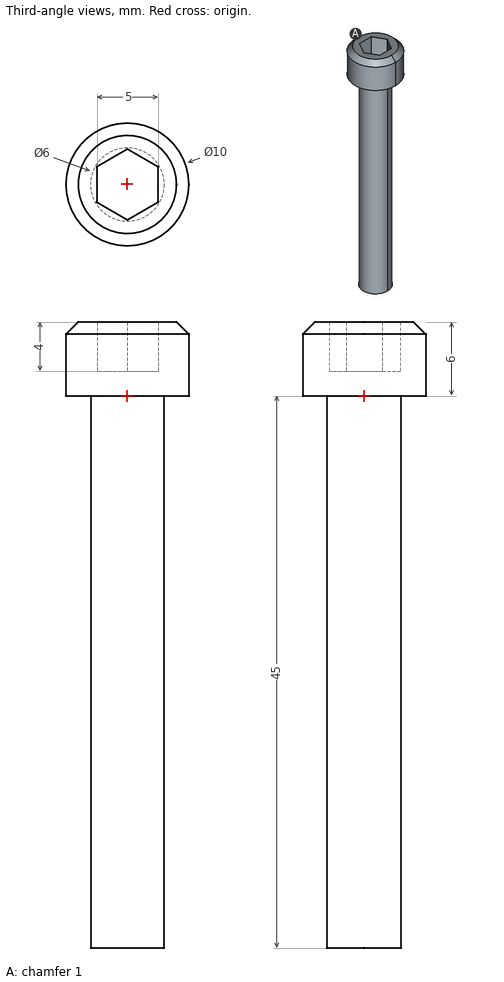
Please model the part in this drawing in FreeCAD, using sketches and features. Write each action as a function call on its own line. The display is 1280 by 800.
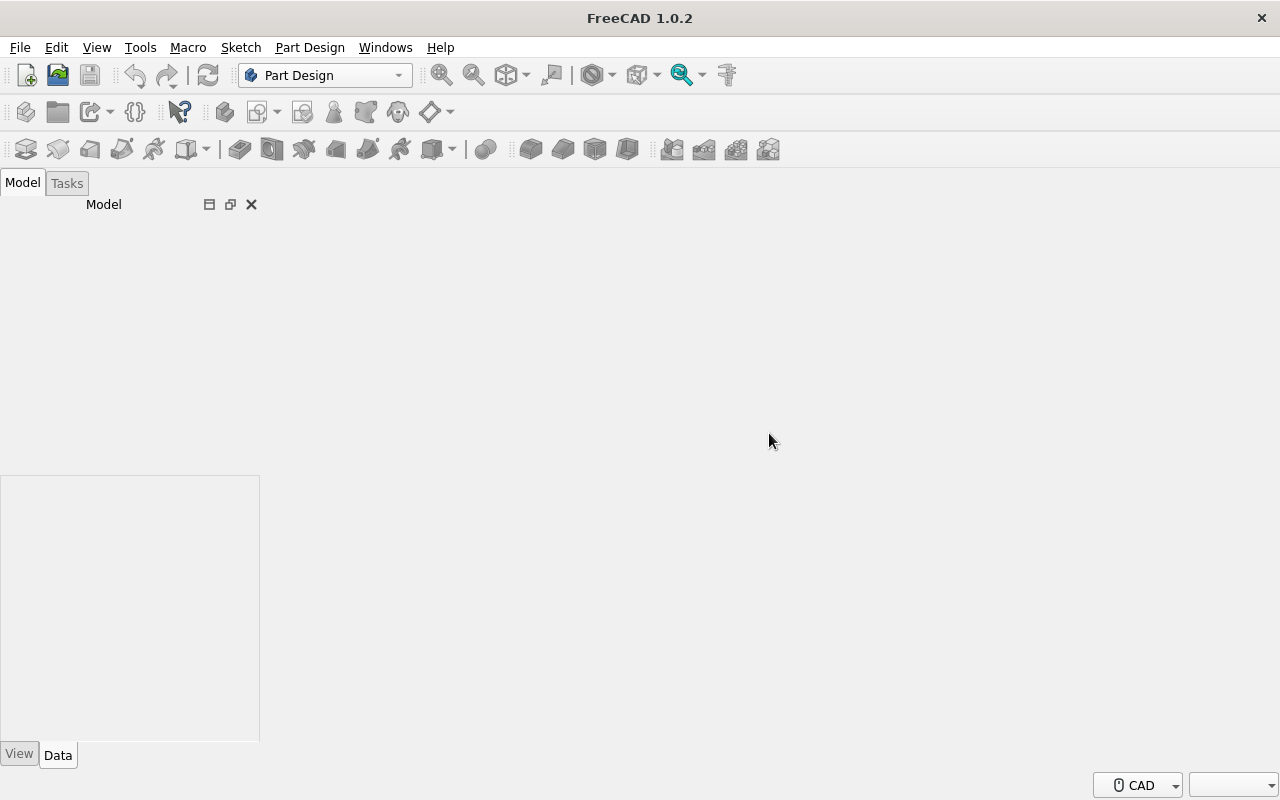
click(26, 76)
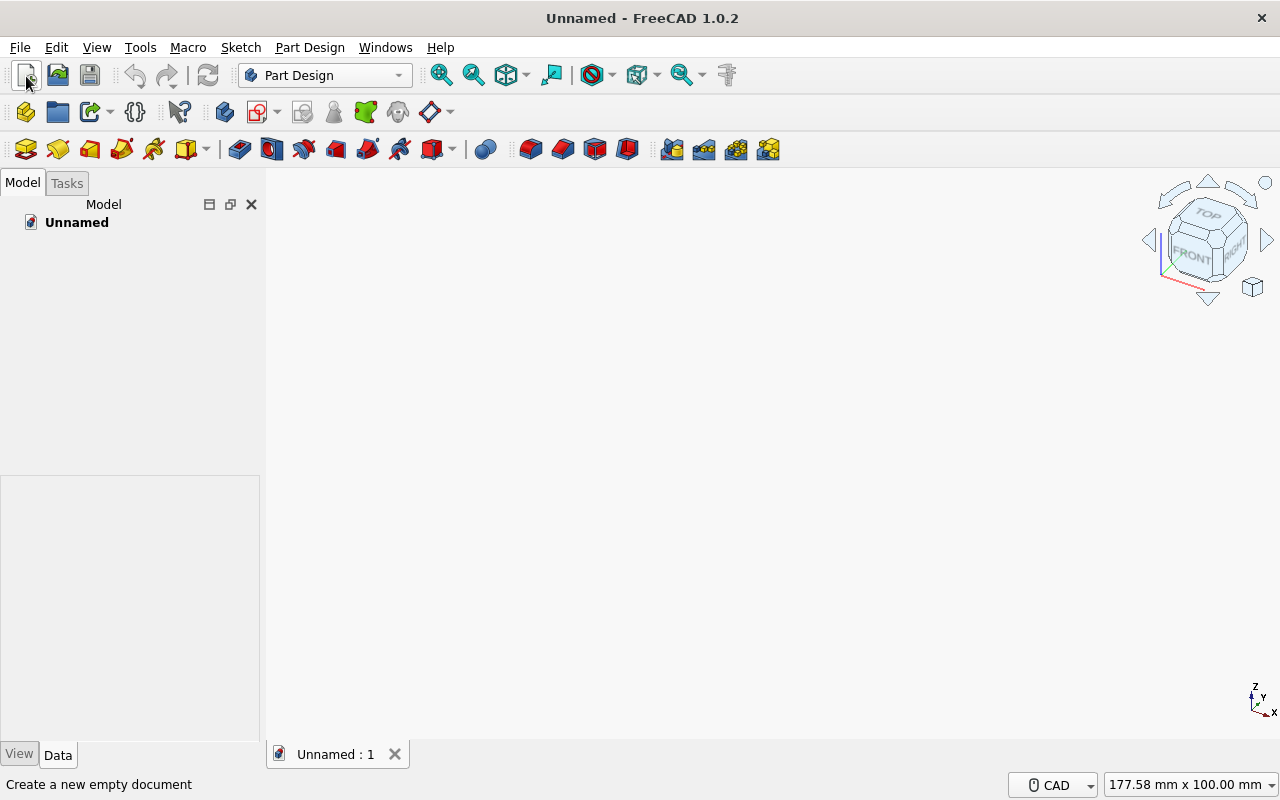
click(258, 112)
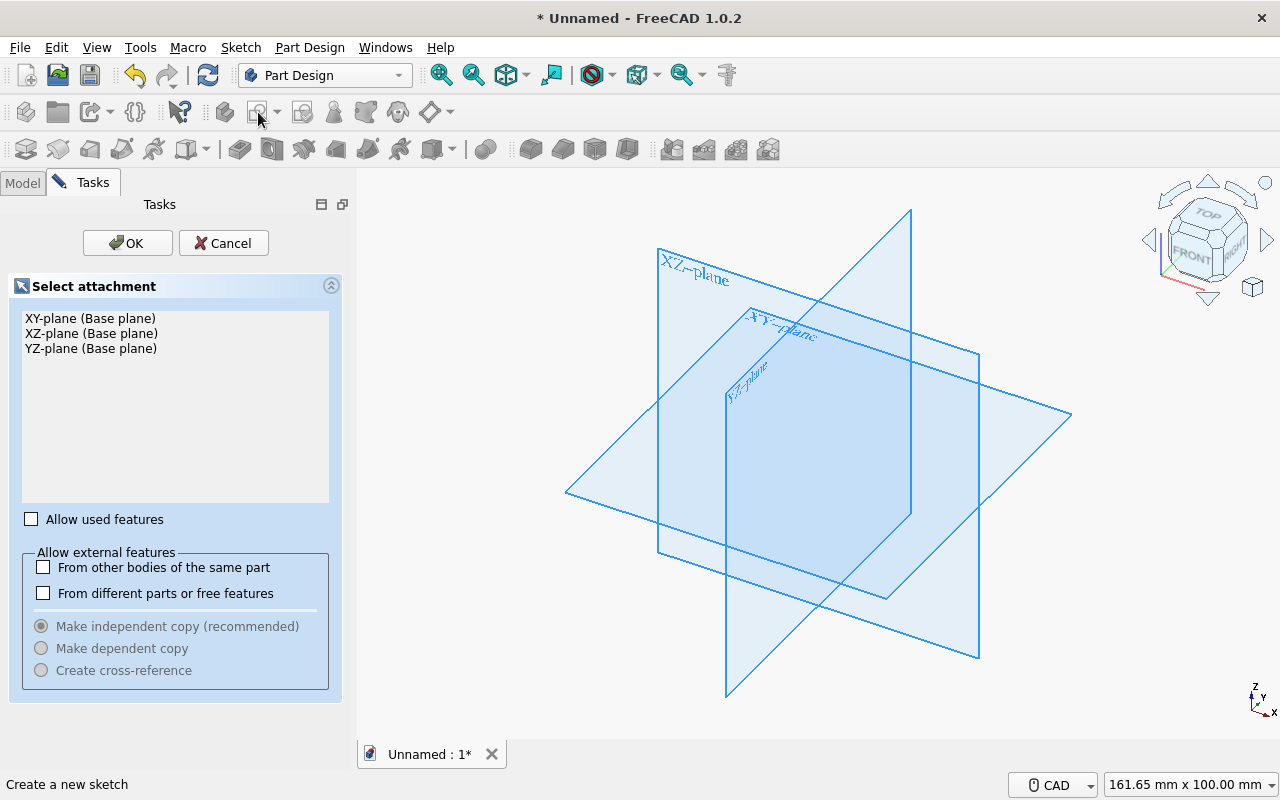
click(82, 318)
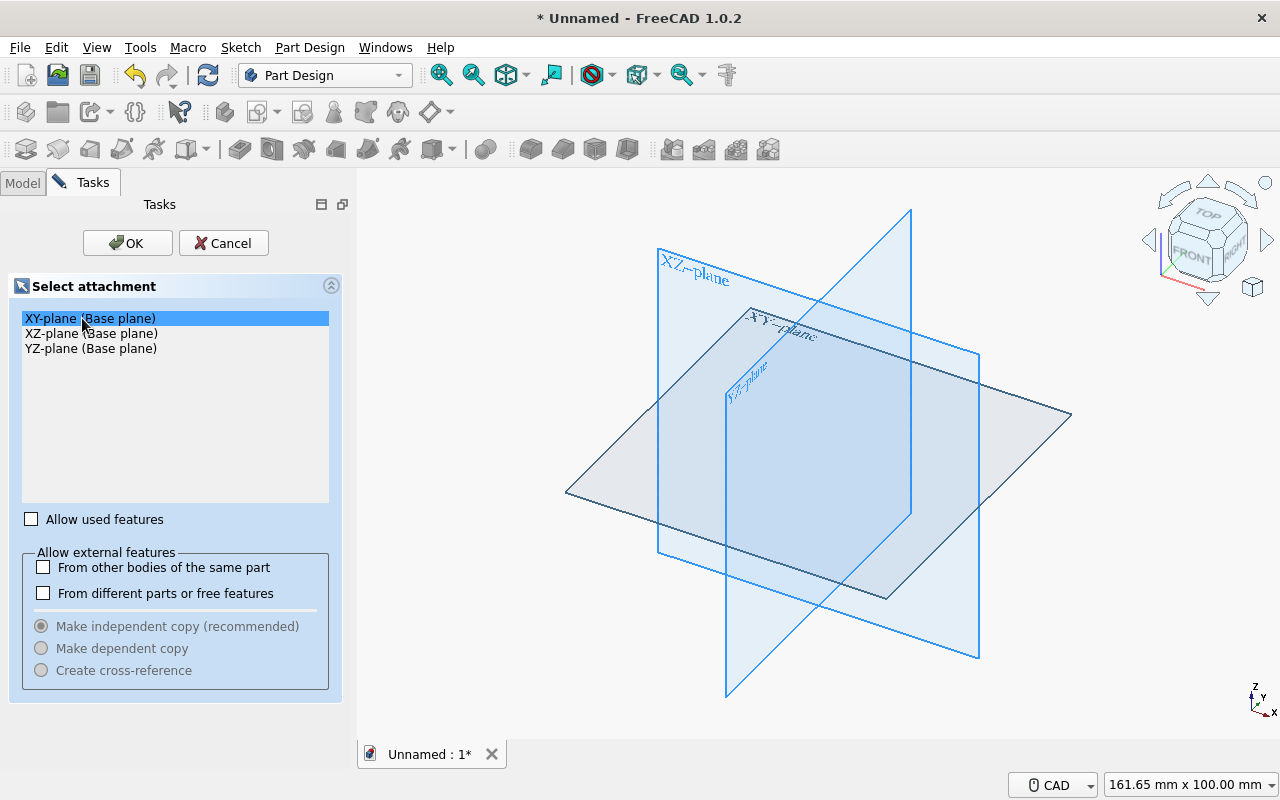
click(128, 243)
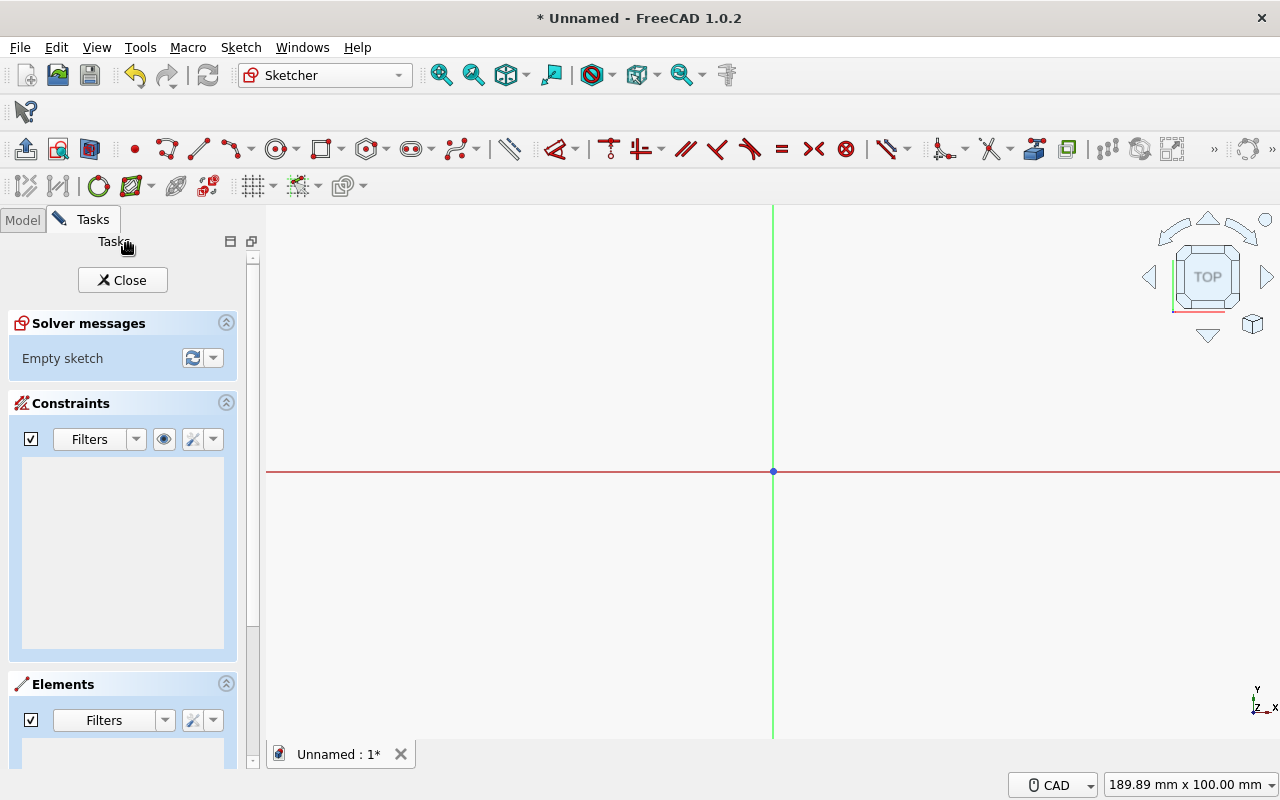
scroll(787, 472, up, 9)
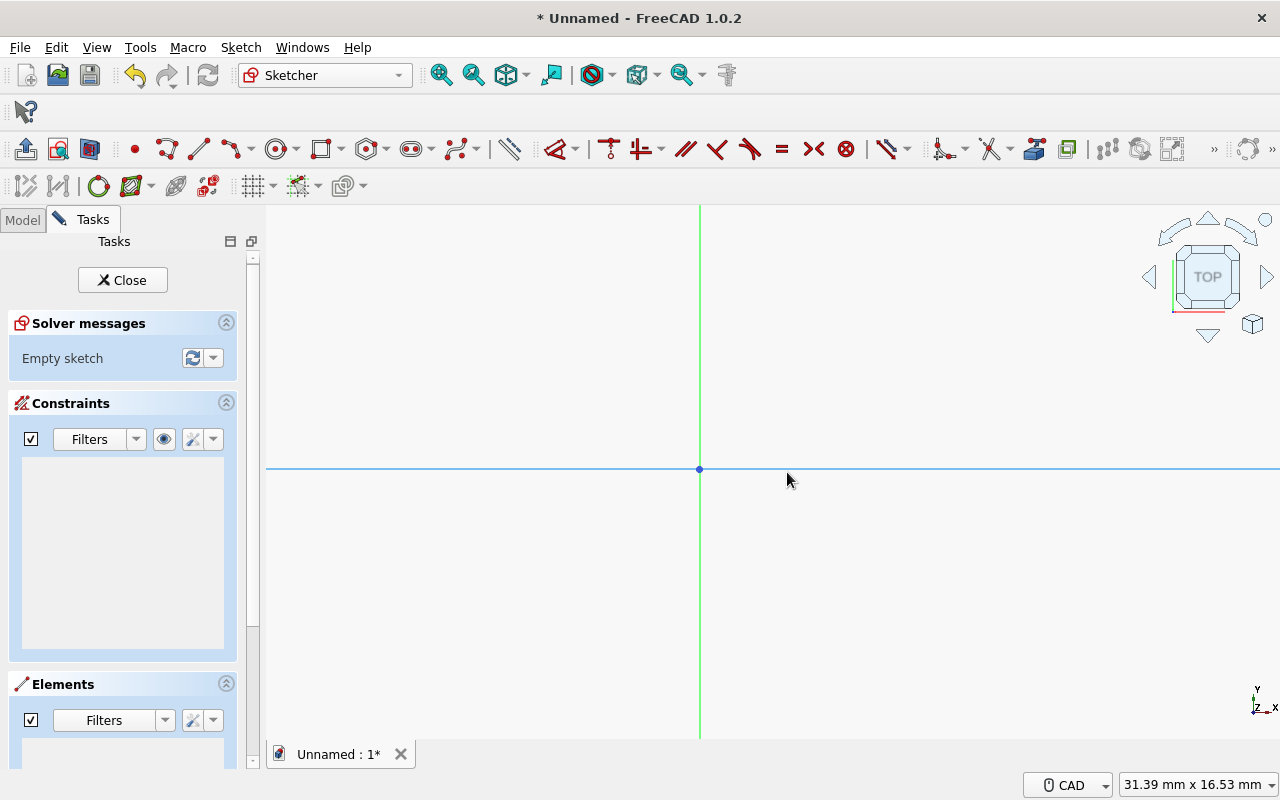
click(276, 150)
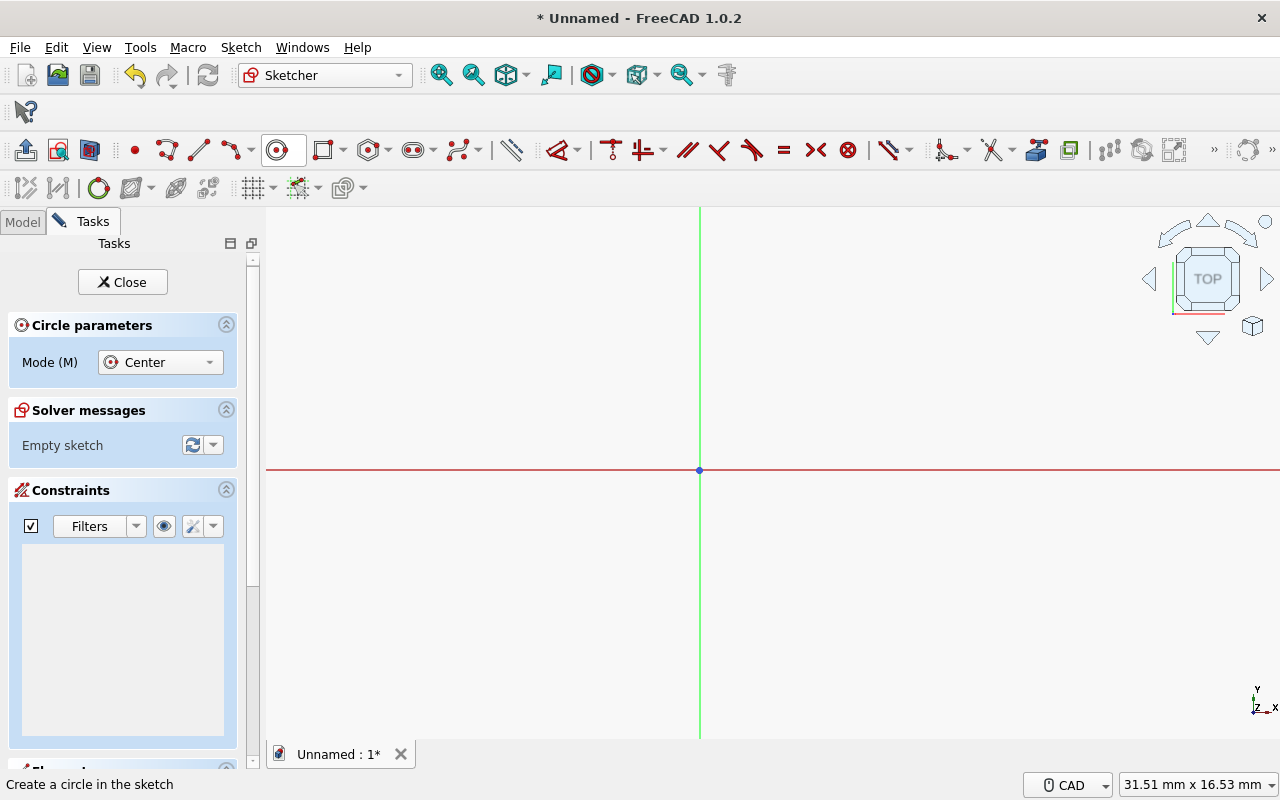
click(700, 470)
move(814, 357)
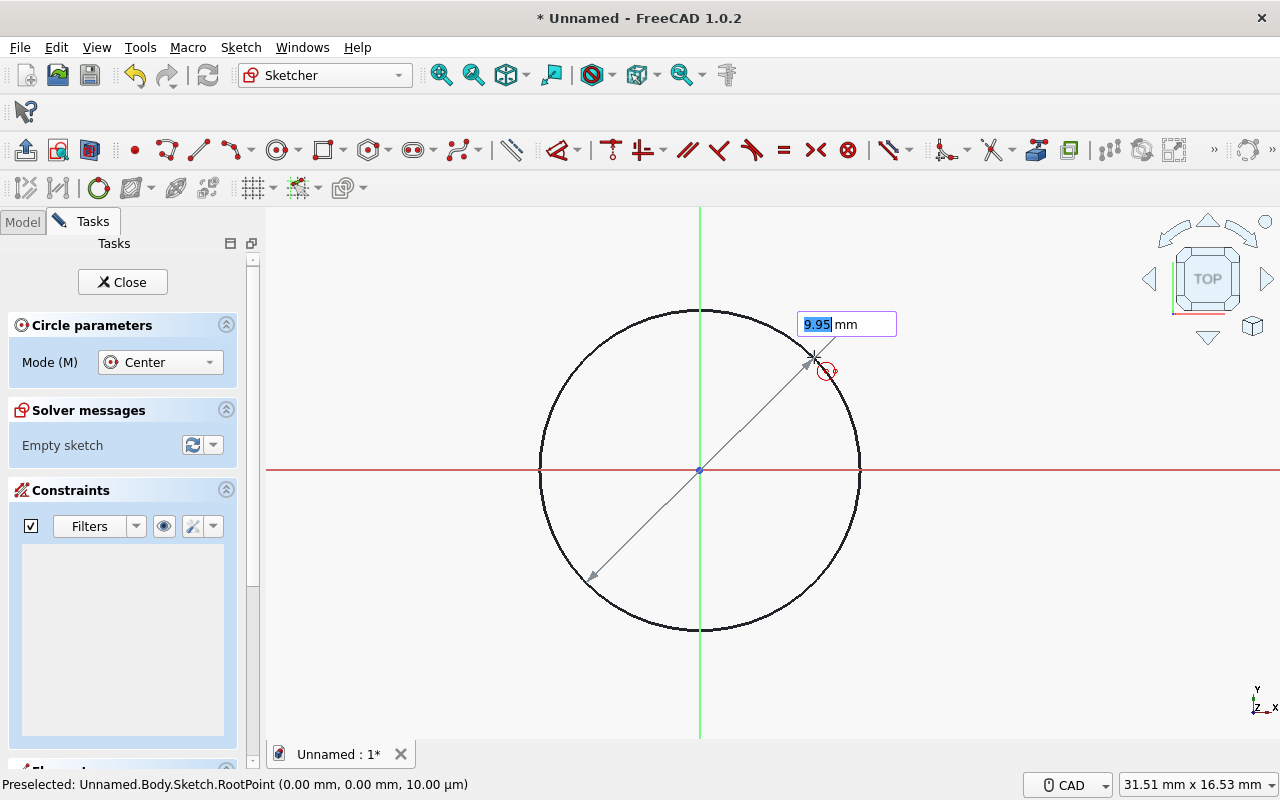
text(10)
key(Return)
key(Escape)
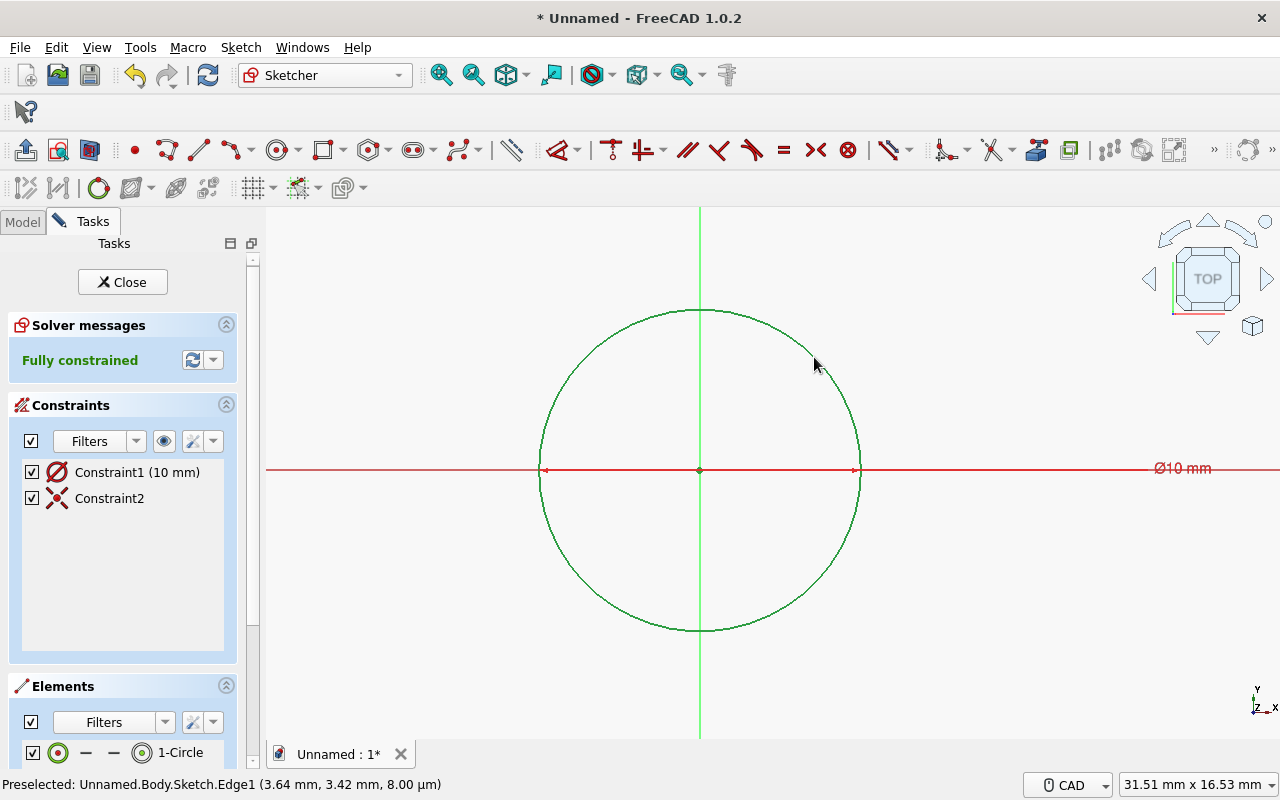
click(123, 282)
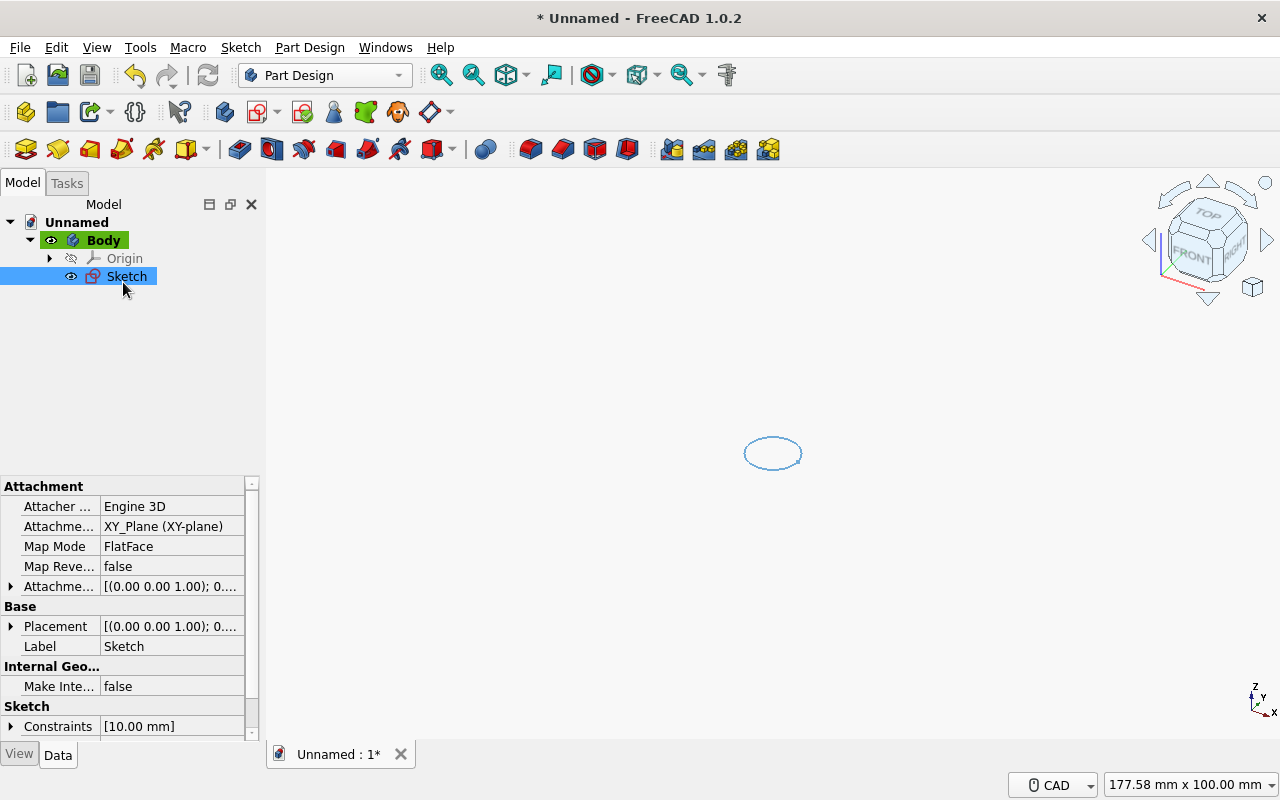
click(26, 150)